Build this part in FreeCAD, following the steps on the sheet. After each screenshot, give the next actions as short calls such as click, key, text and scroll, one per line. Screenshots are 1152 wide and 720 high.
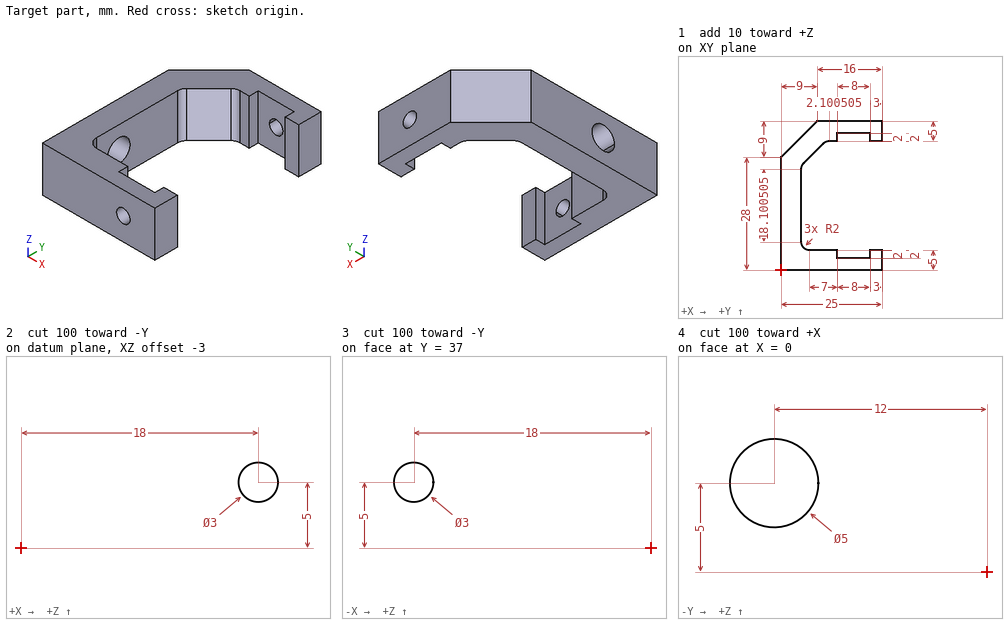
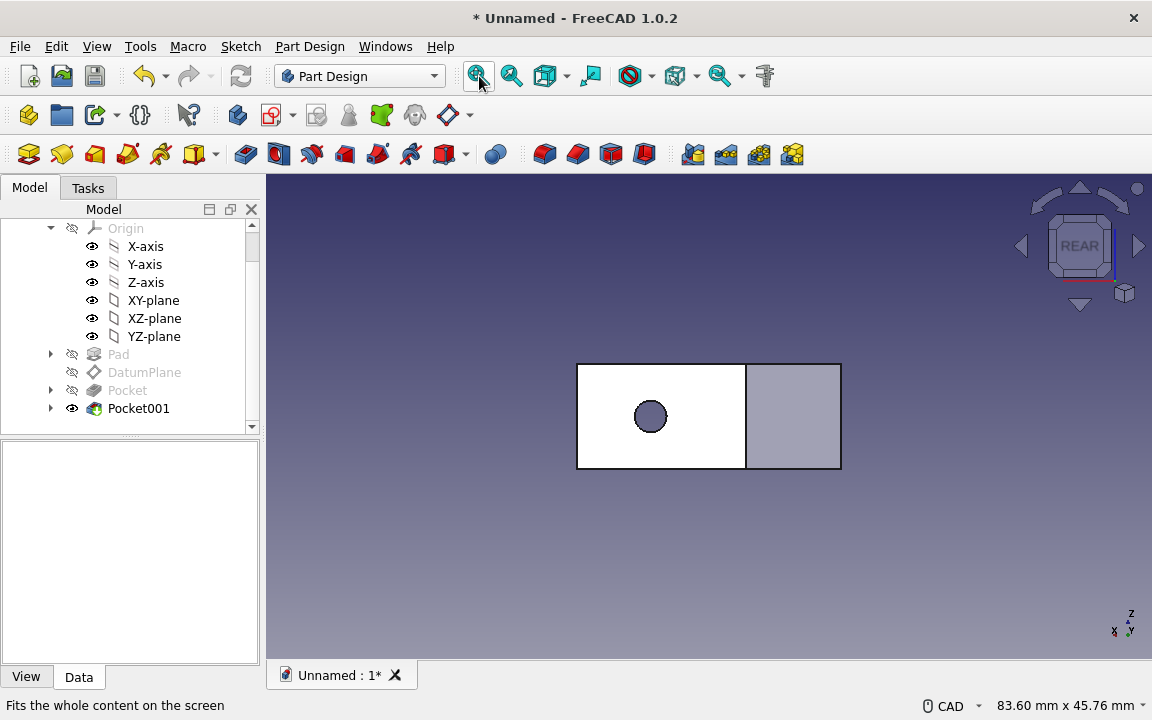
key(6)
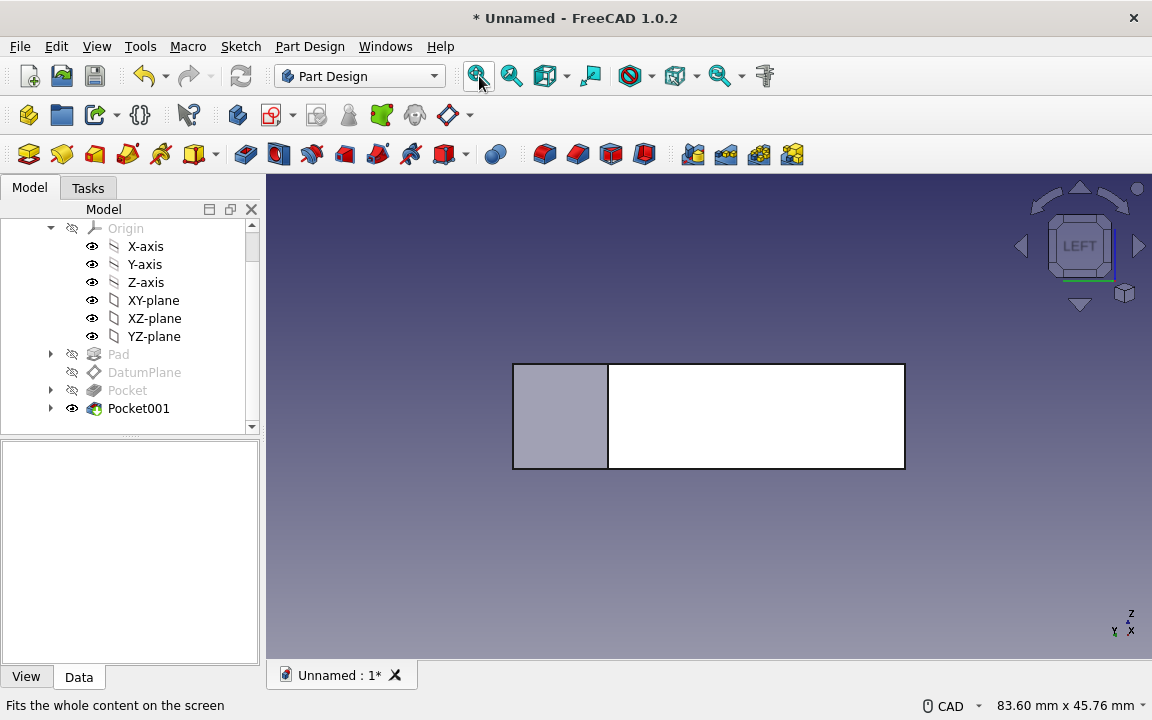
key(v)
key(f)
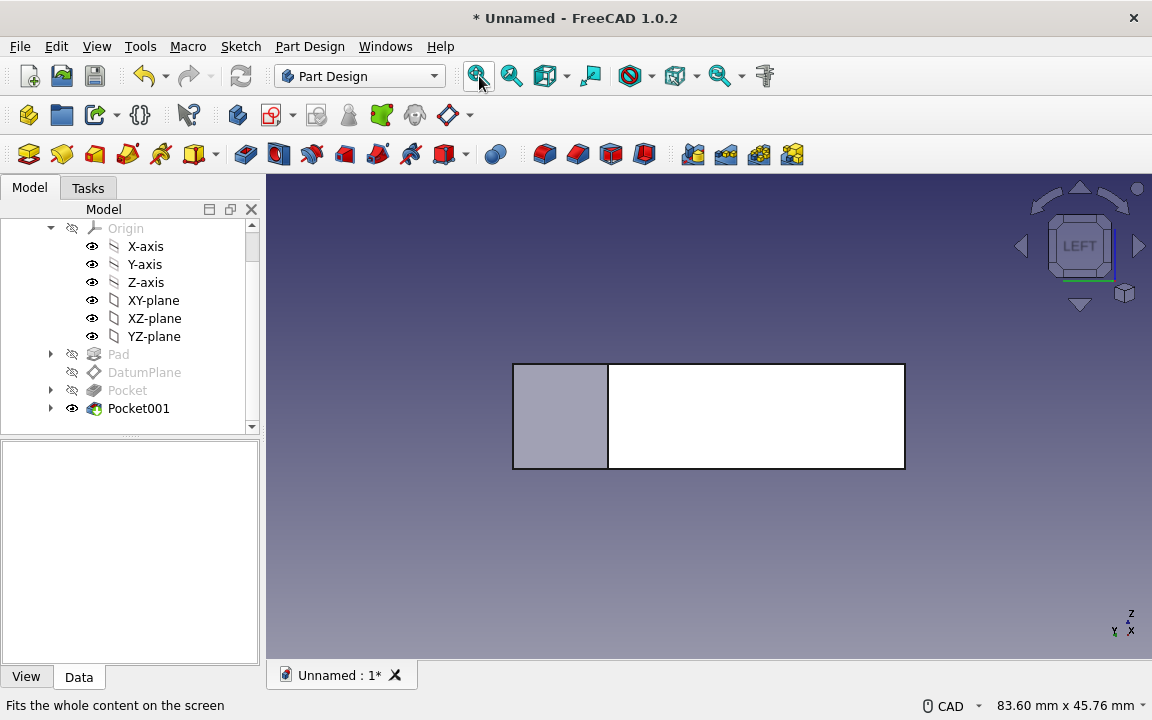
click(672, 415)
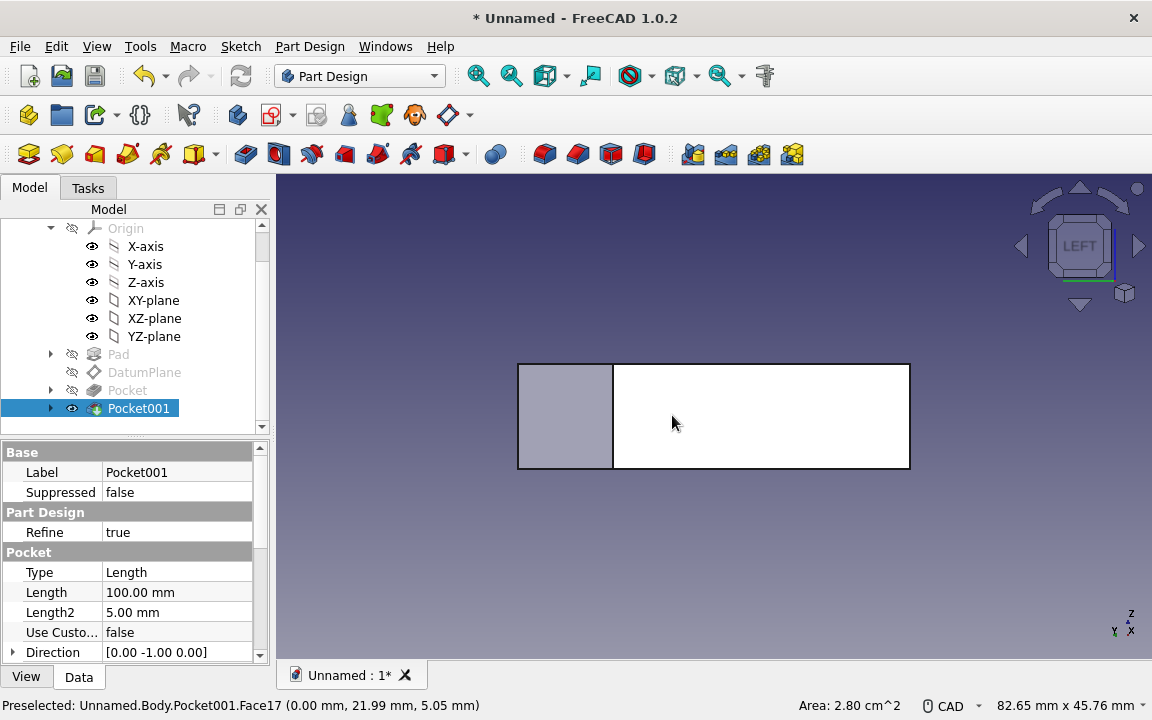
click(270, 116)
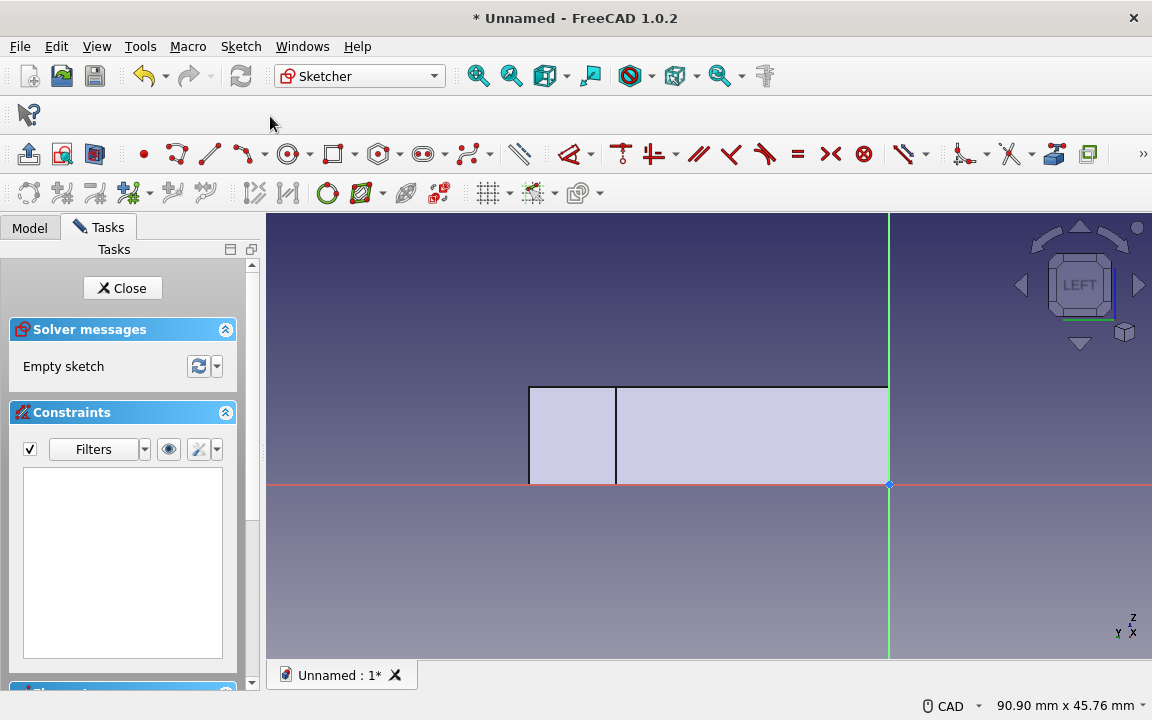
scroll(798, 436, up, 9)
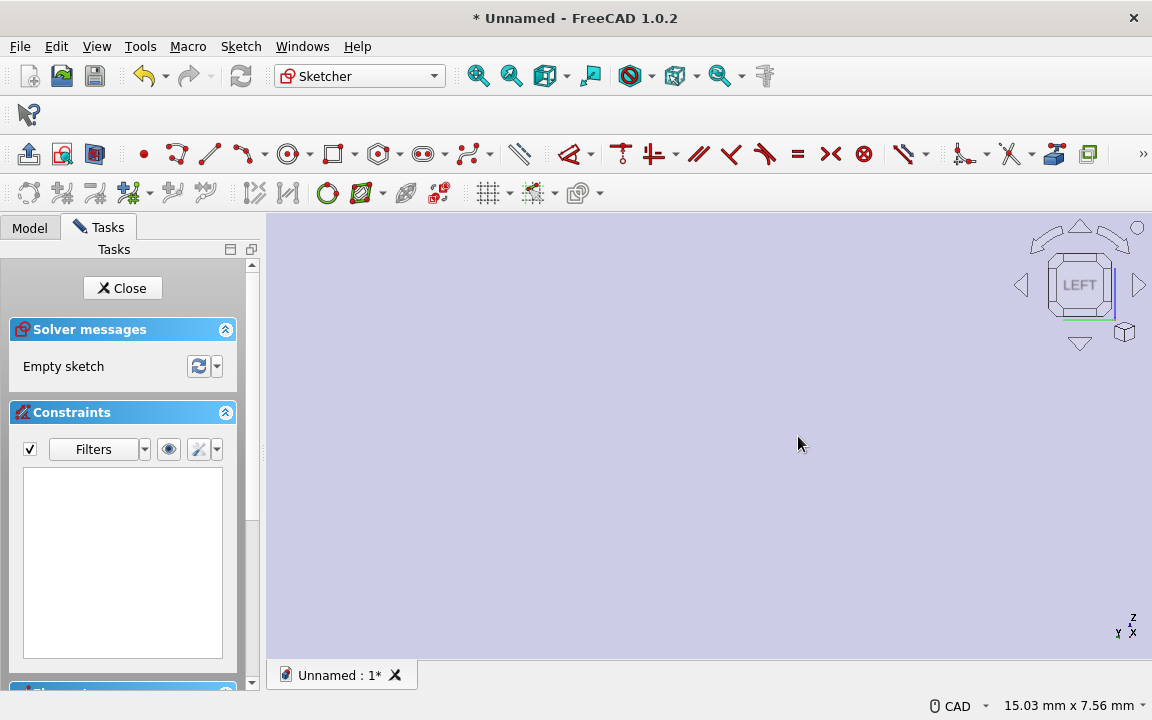
key(g)
key(c)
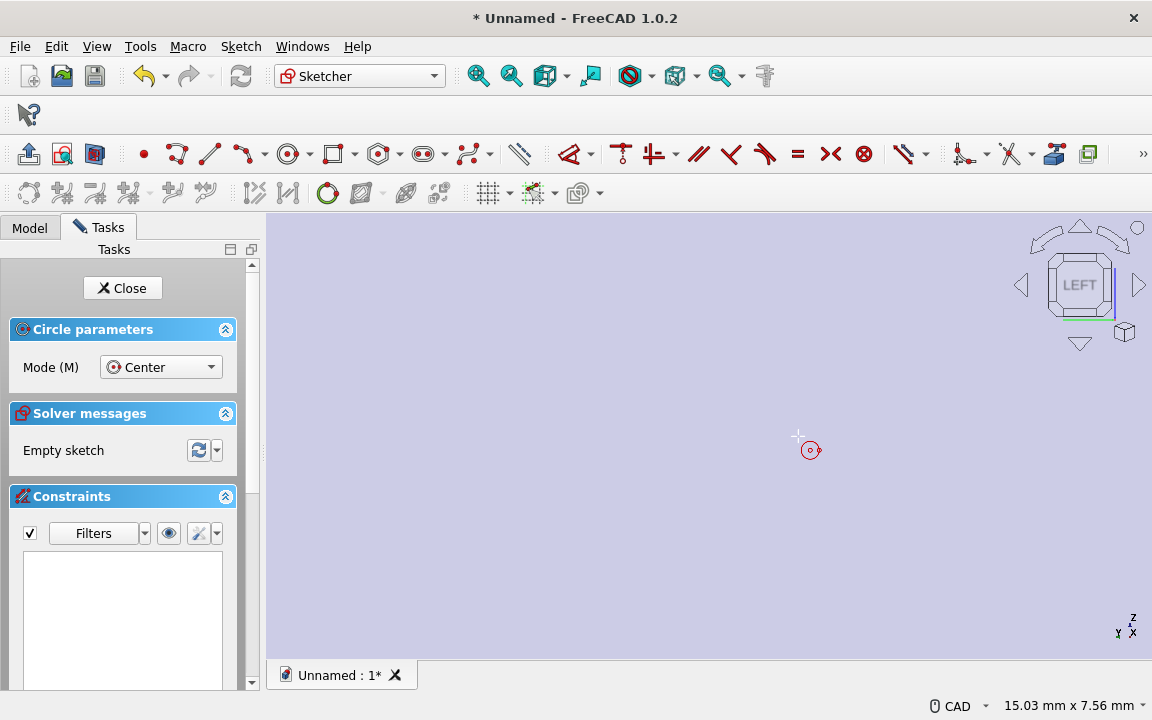
click(640, 433)
click(744, 329)
key(Escape)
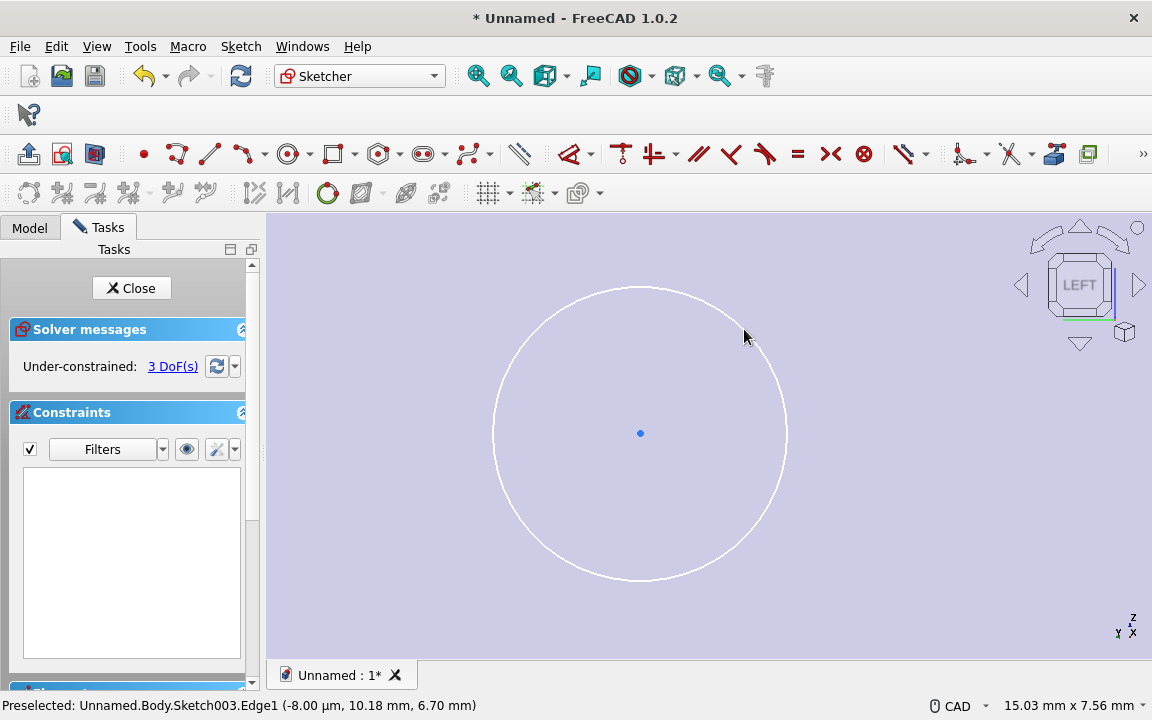
key(d)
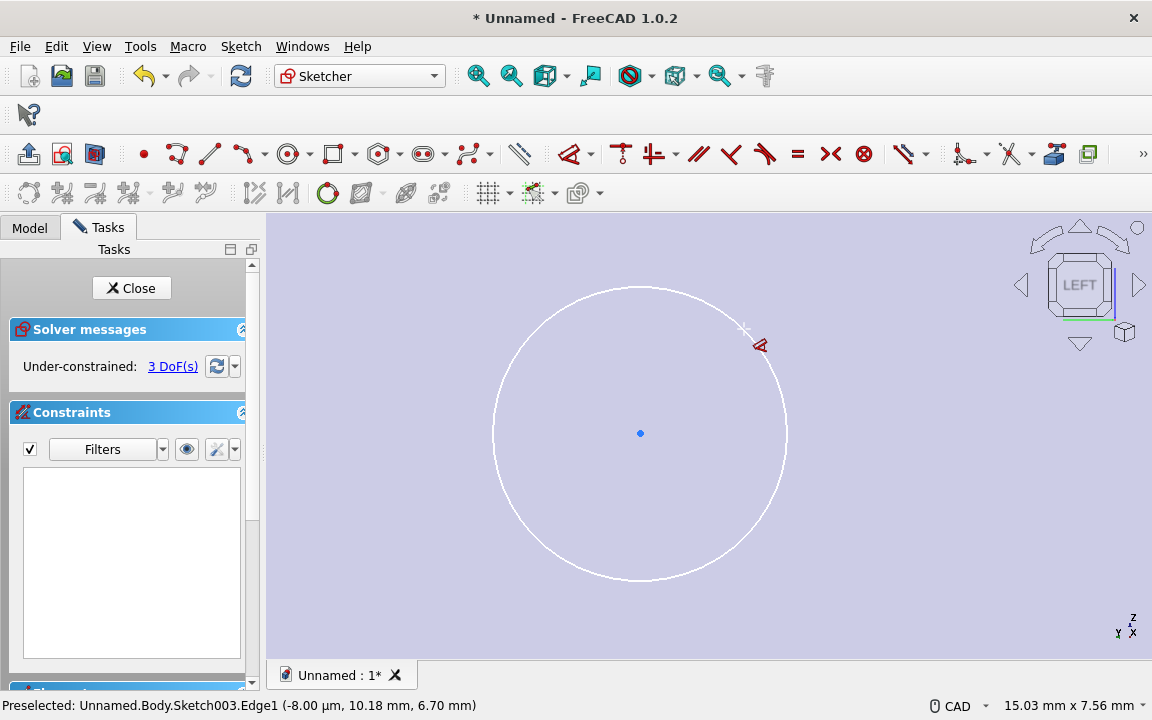
click(744, 330)
click(767, 307)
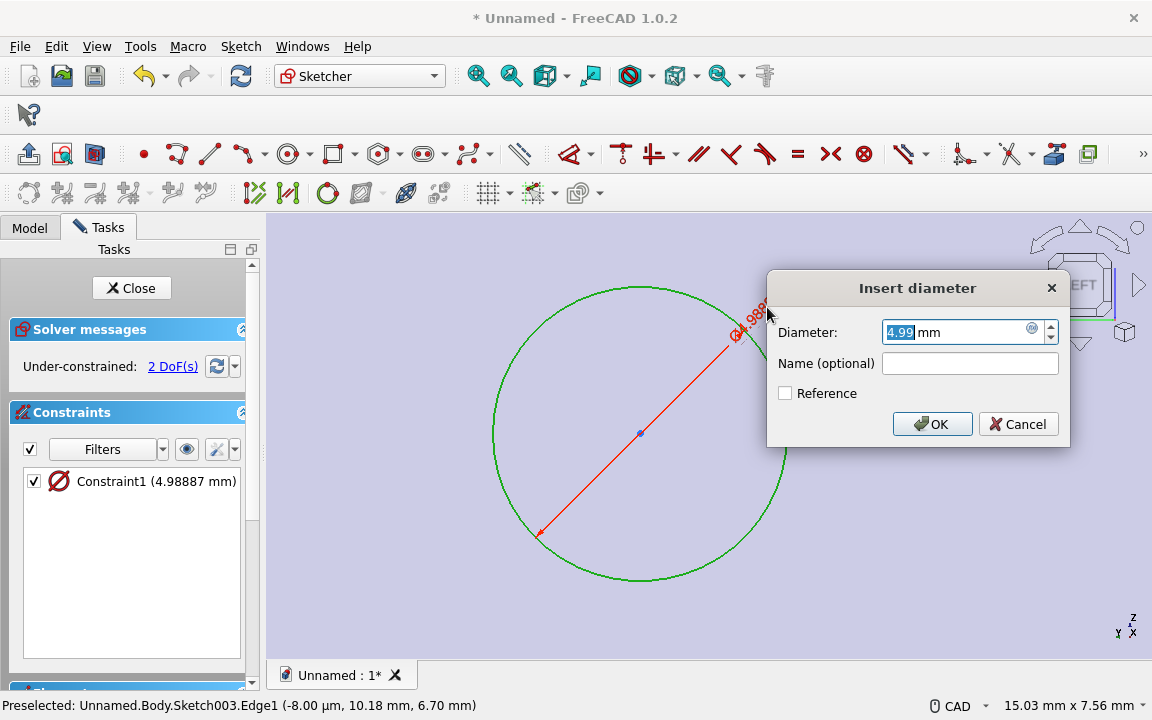
text(5)
key(Return)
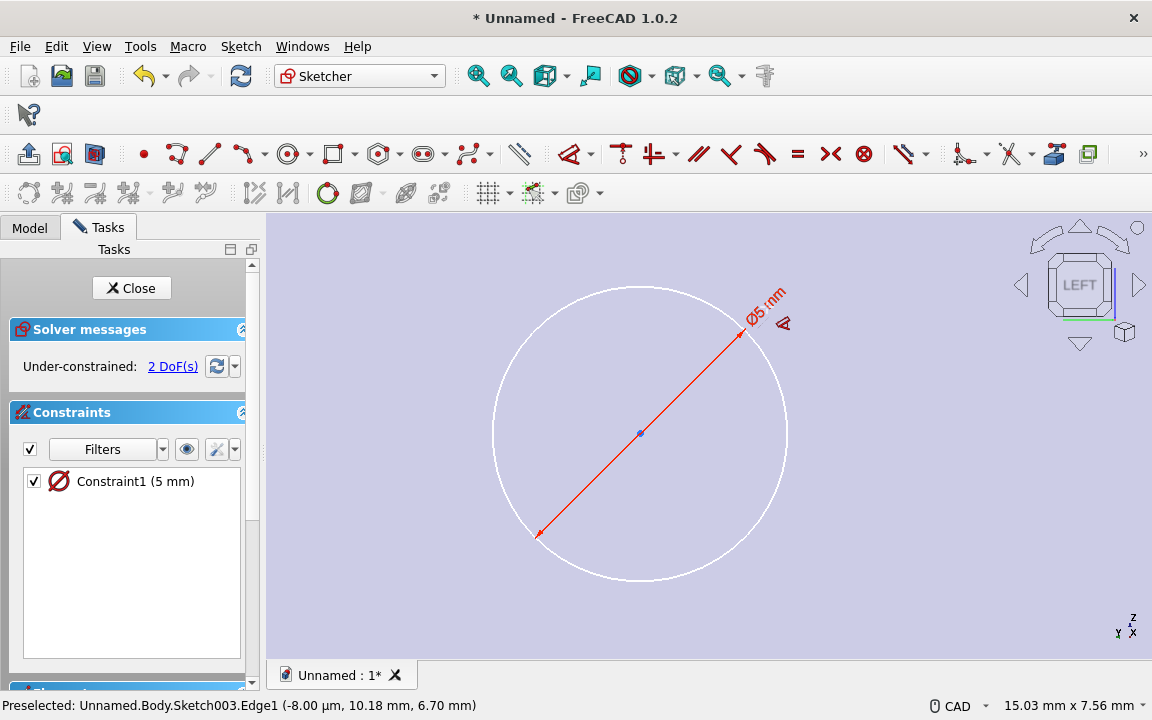
click(640, 434)
click(606, 532)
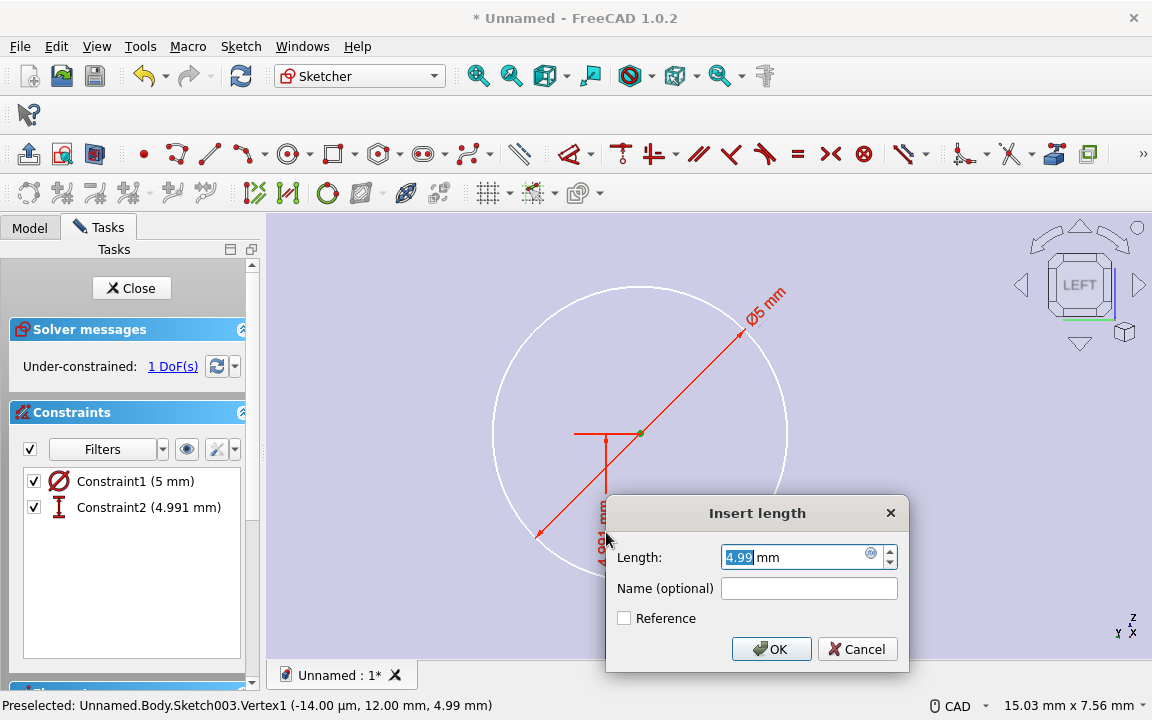
text(5)
key(Return)